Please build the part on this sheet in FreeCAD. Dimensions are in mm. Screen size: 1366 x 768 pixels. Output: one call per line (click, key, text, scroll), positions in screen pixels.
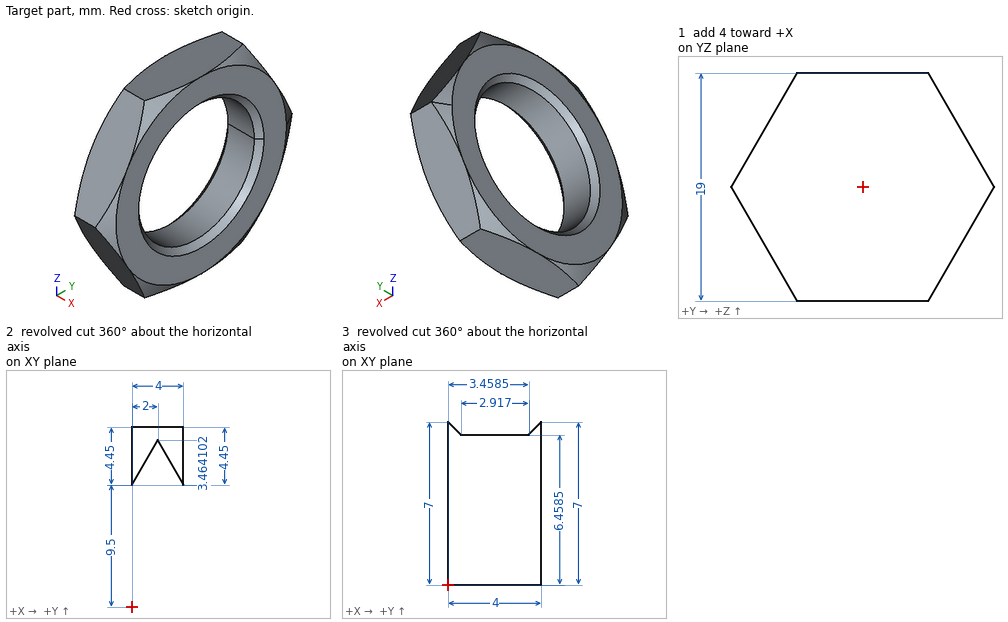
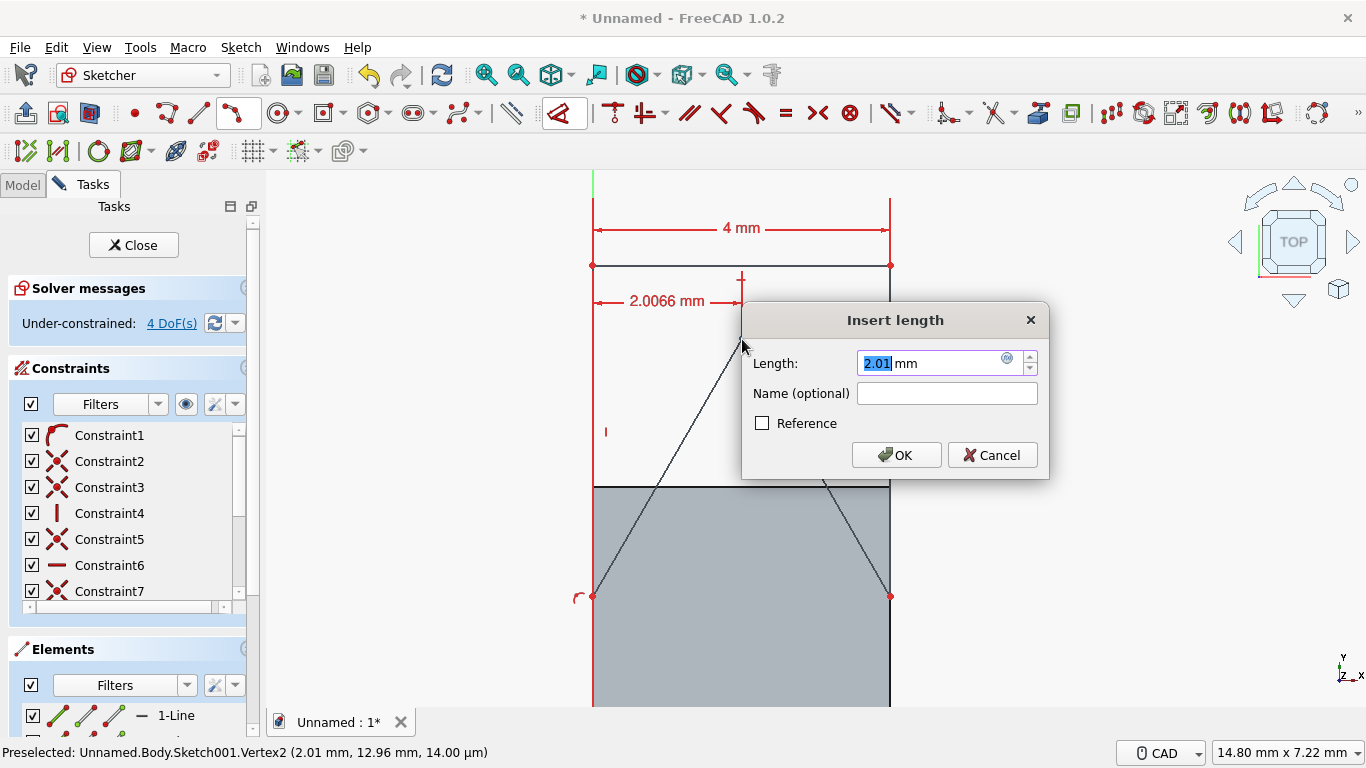
text(2)
key(Return)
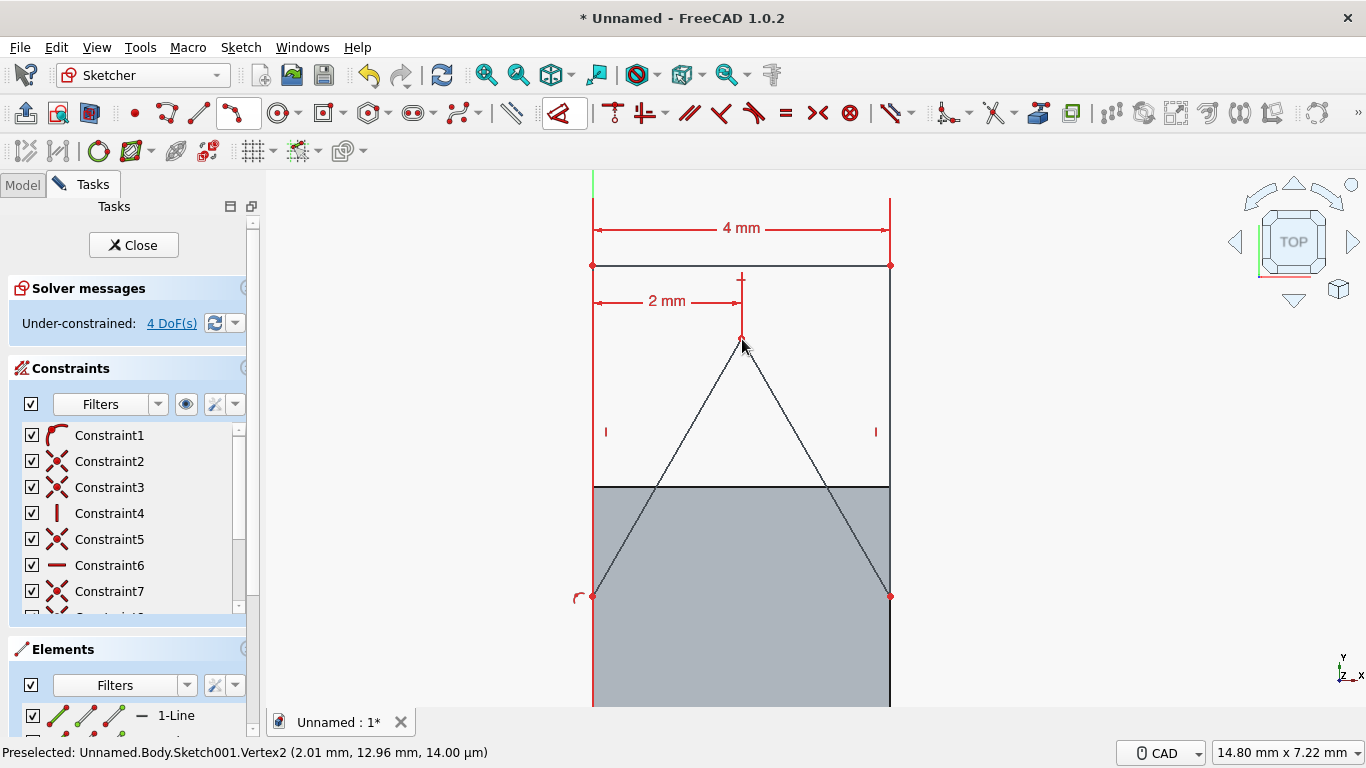
click(890, 498)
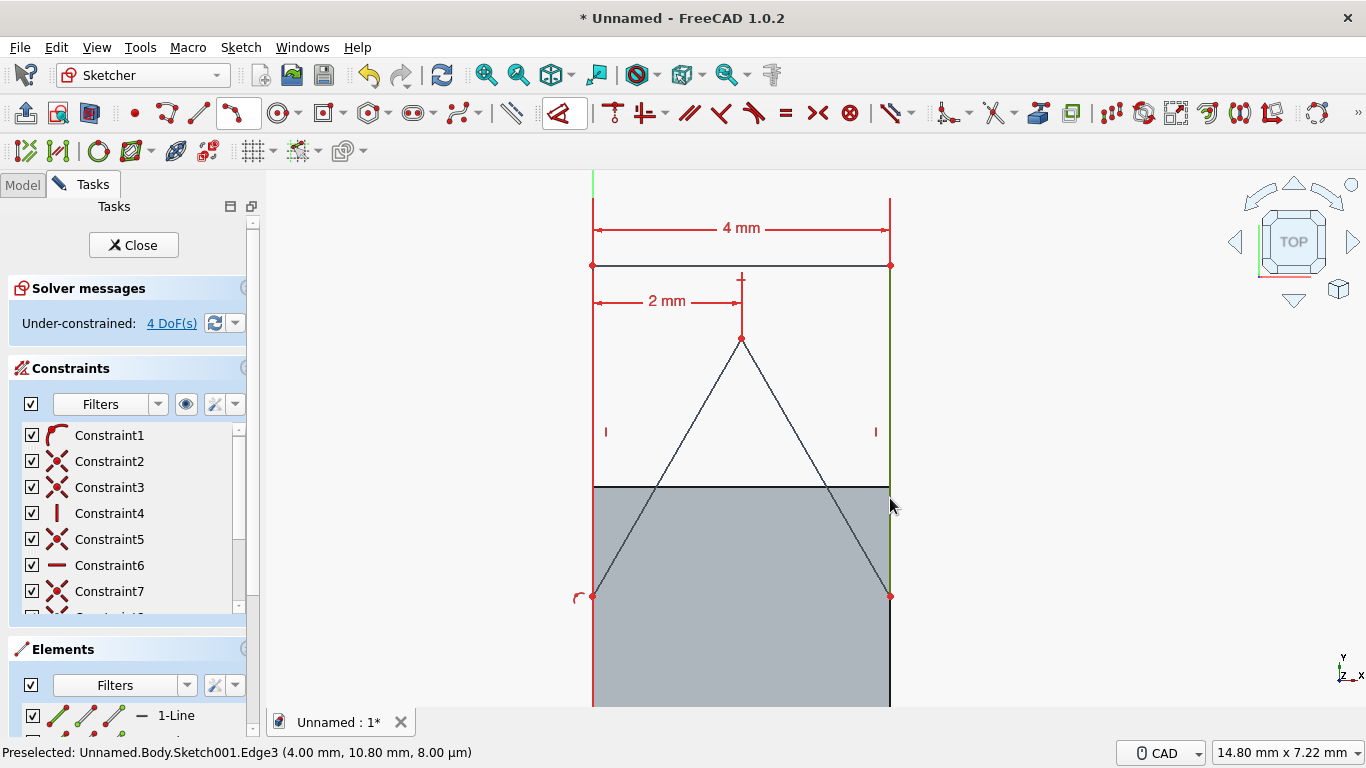
key(i)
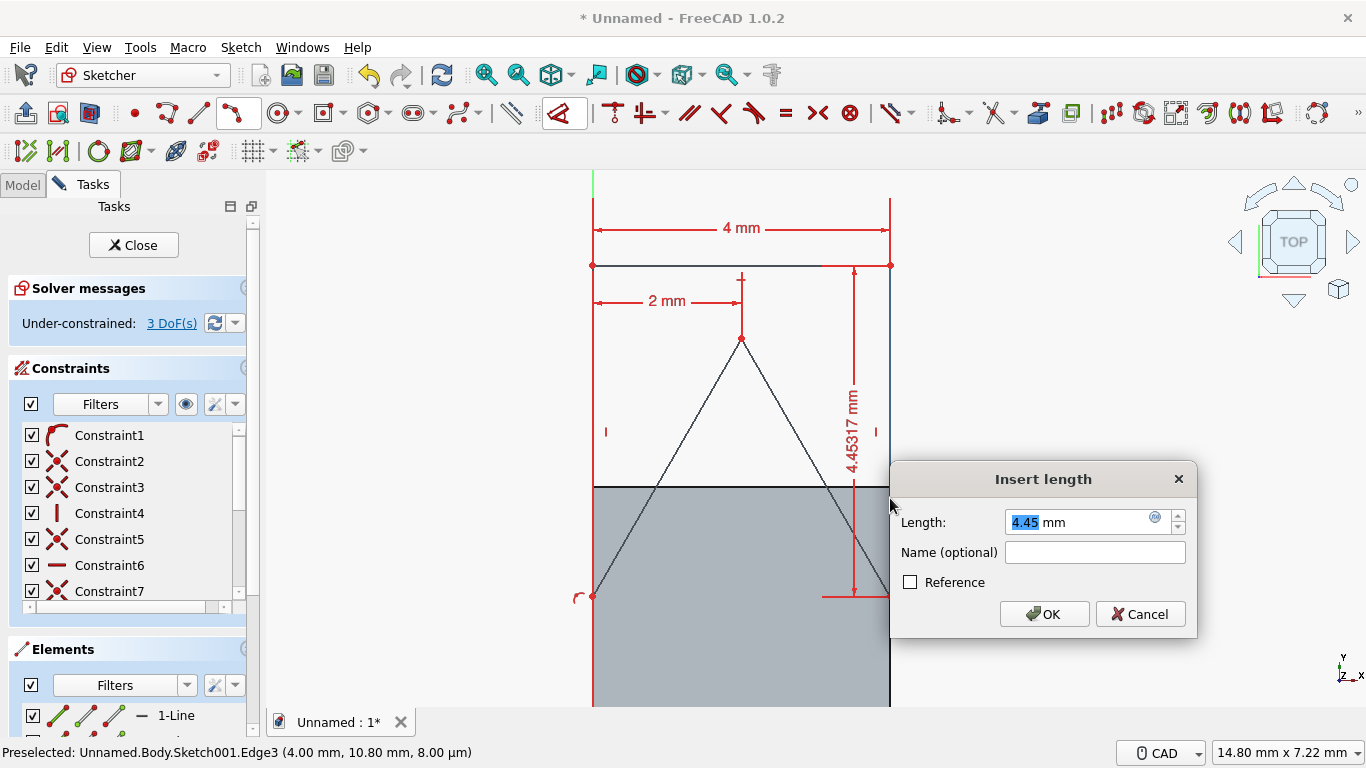
text(4.45)
key(Return)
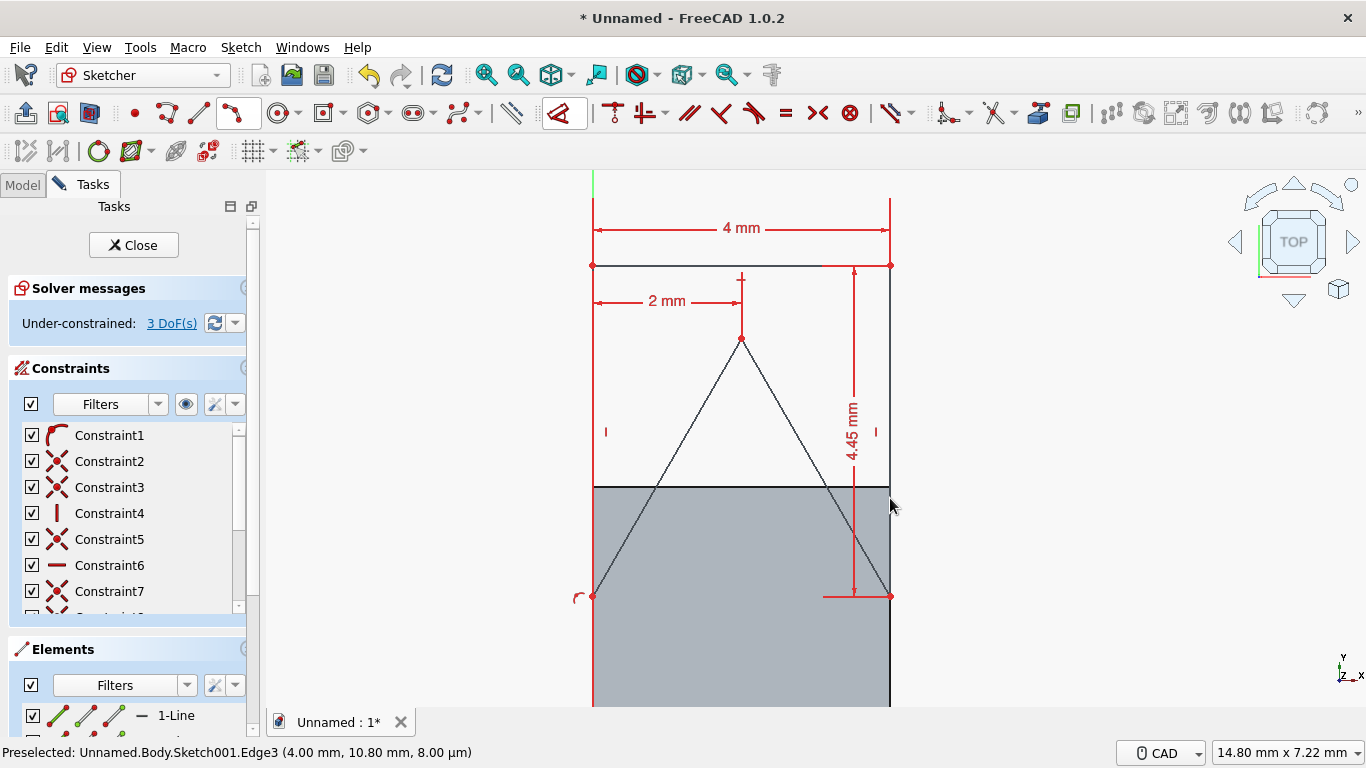
click(593, 365)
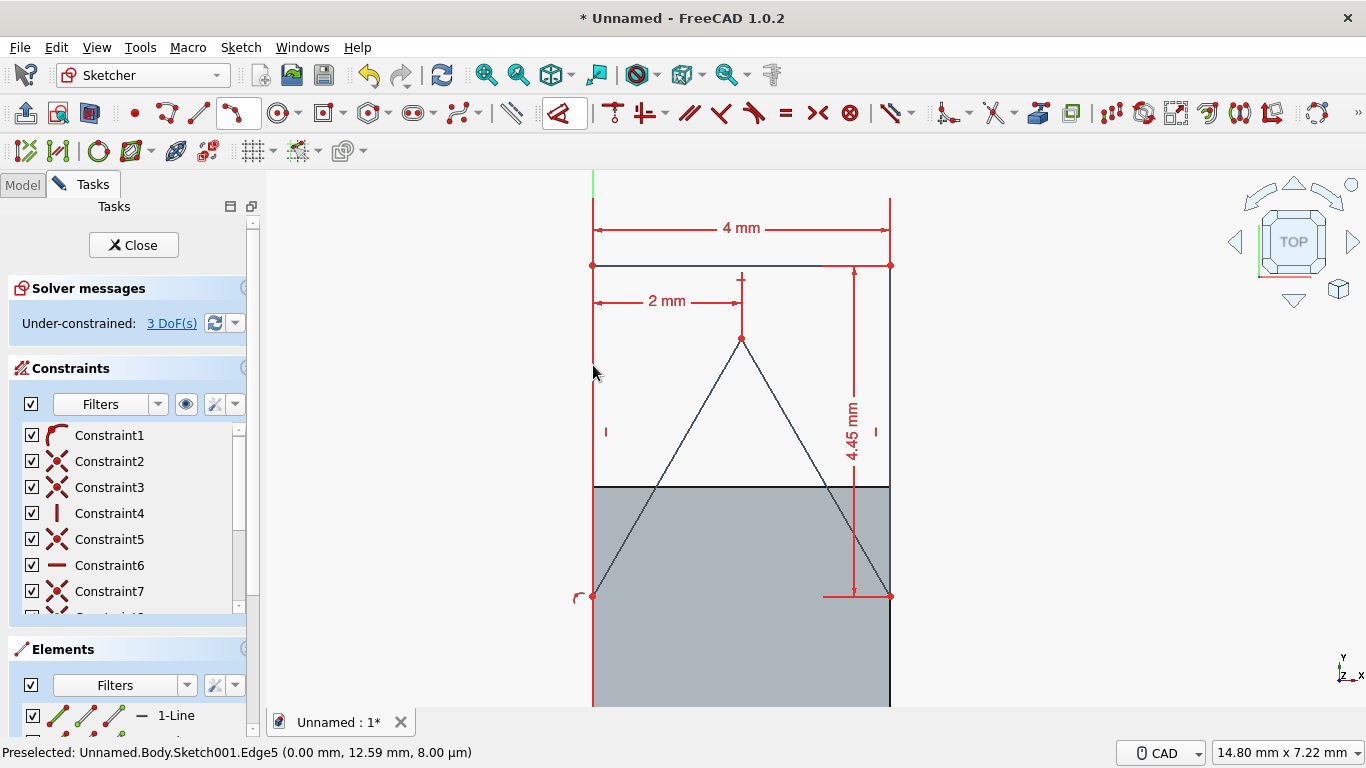
key(i)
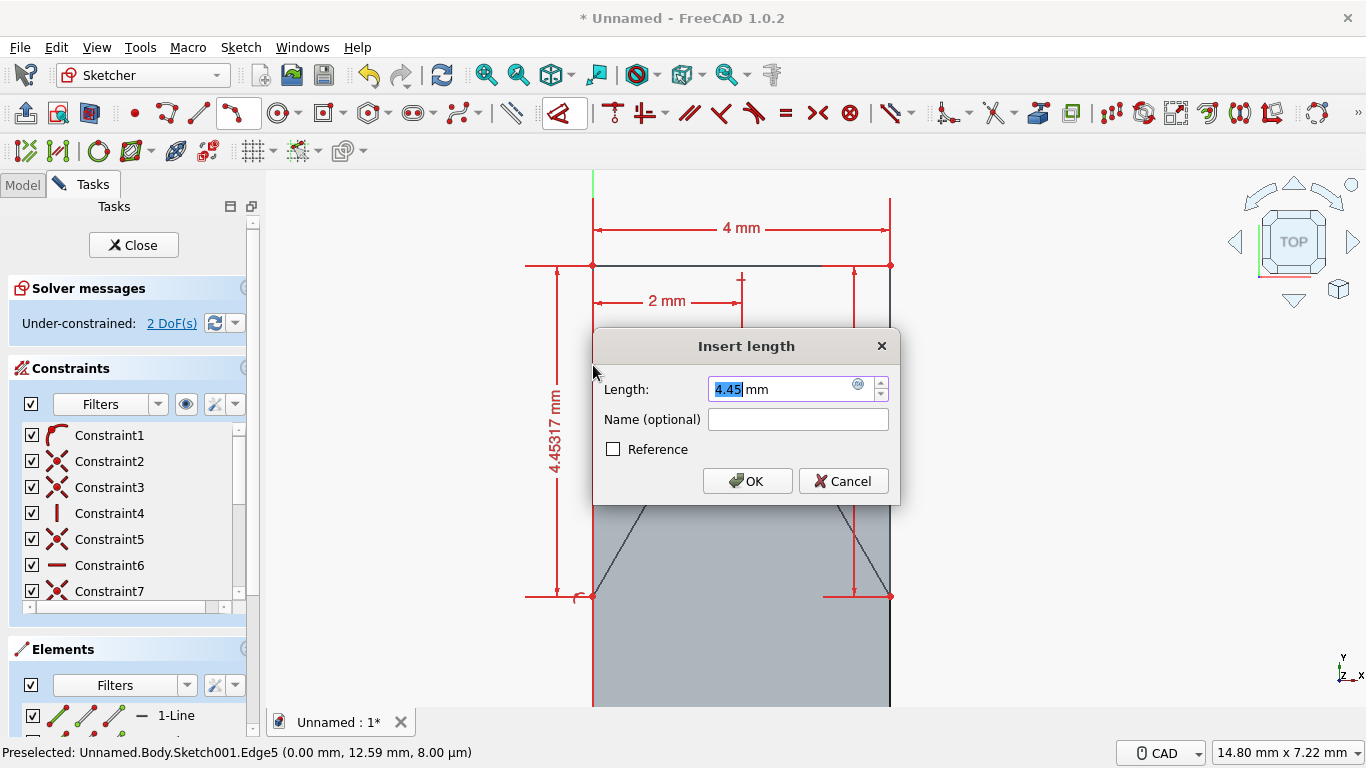
text(4.45)
key(Return)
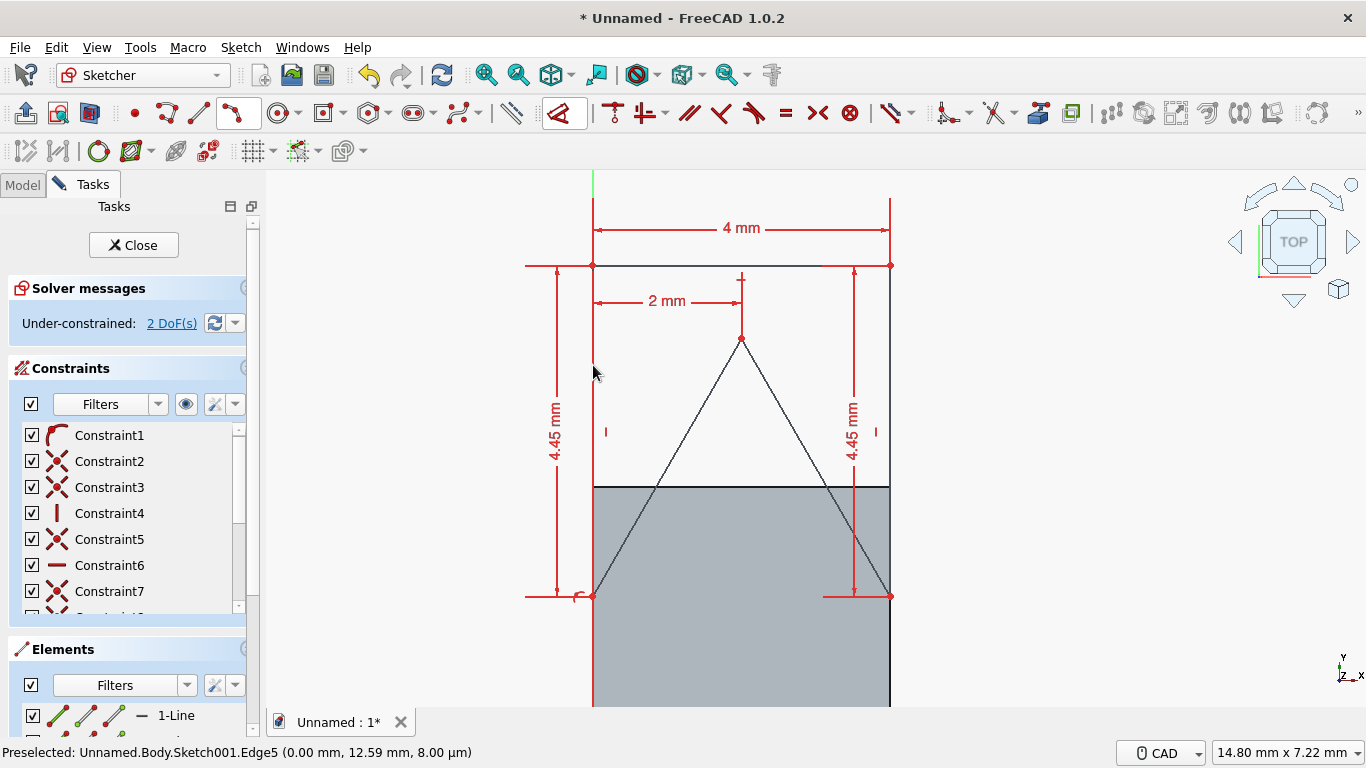
click(593, 597)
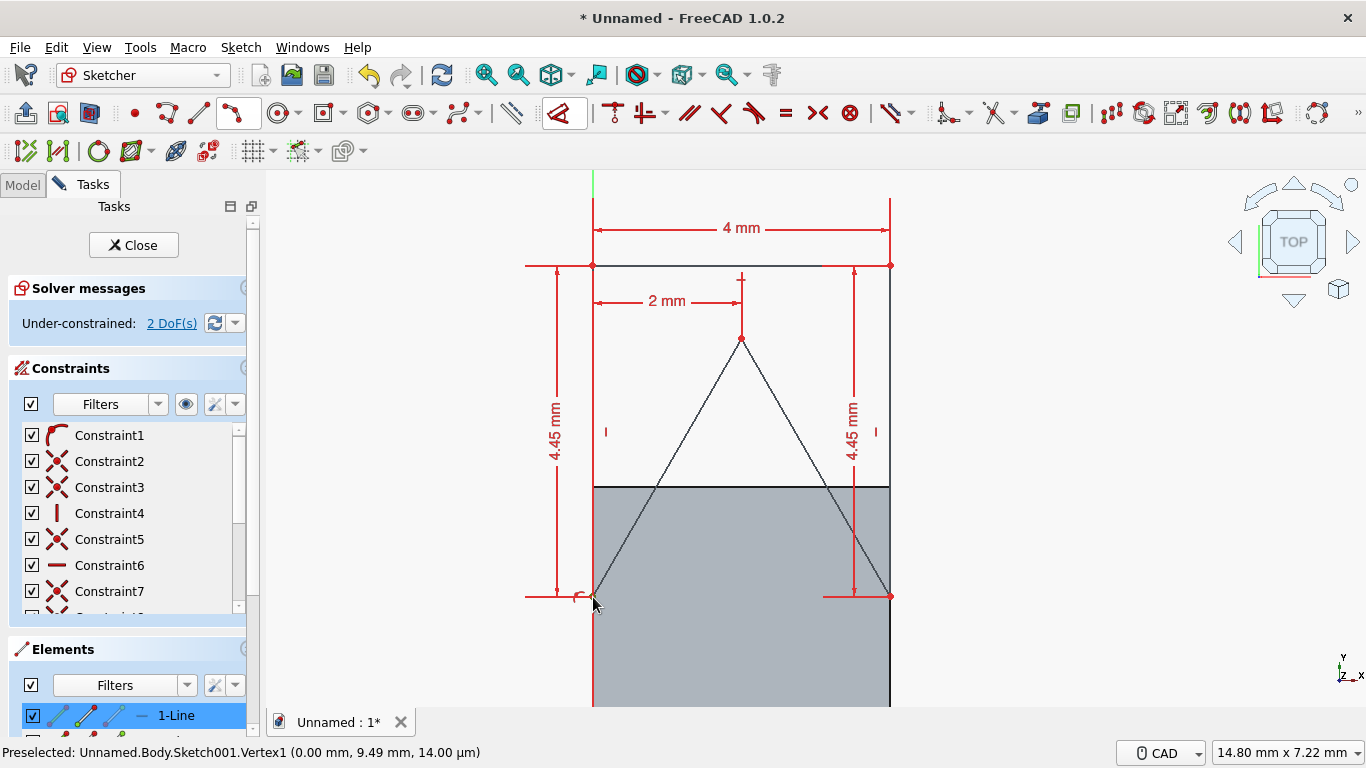
key(i)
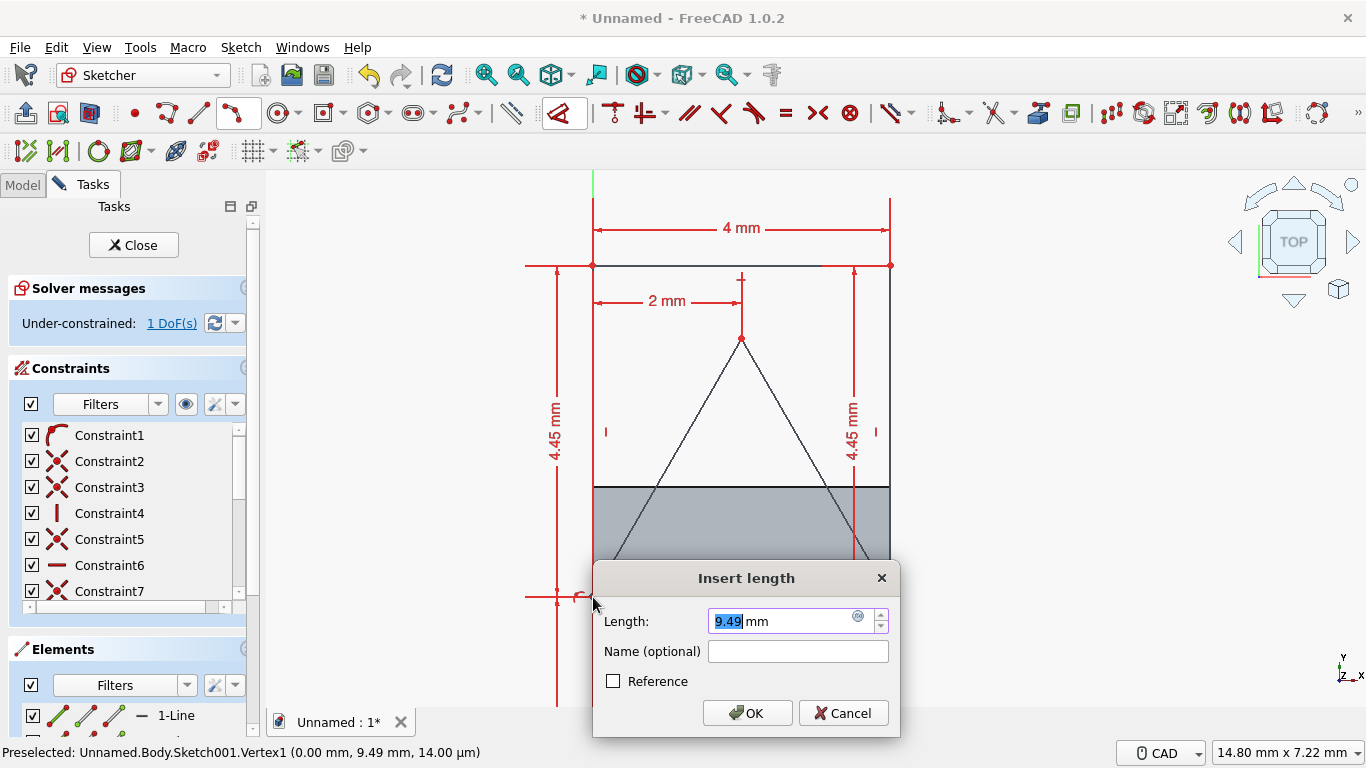
text(9.5)
key(Return)